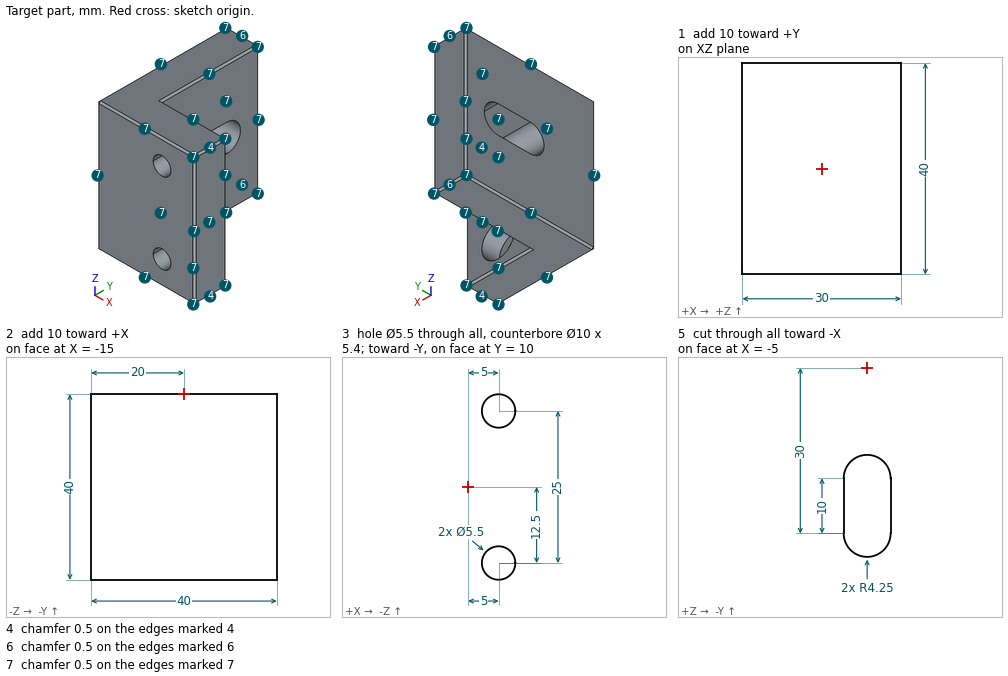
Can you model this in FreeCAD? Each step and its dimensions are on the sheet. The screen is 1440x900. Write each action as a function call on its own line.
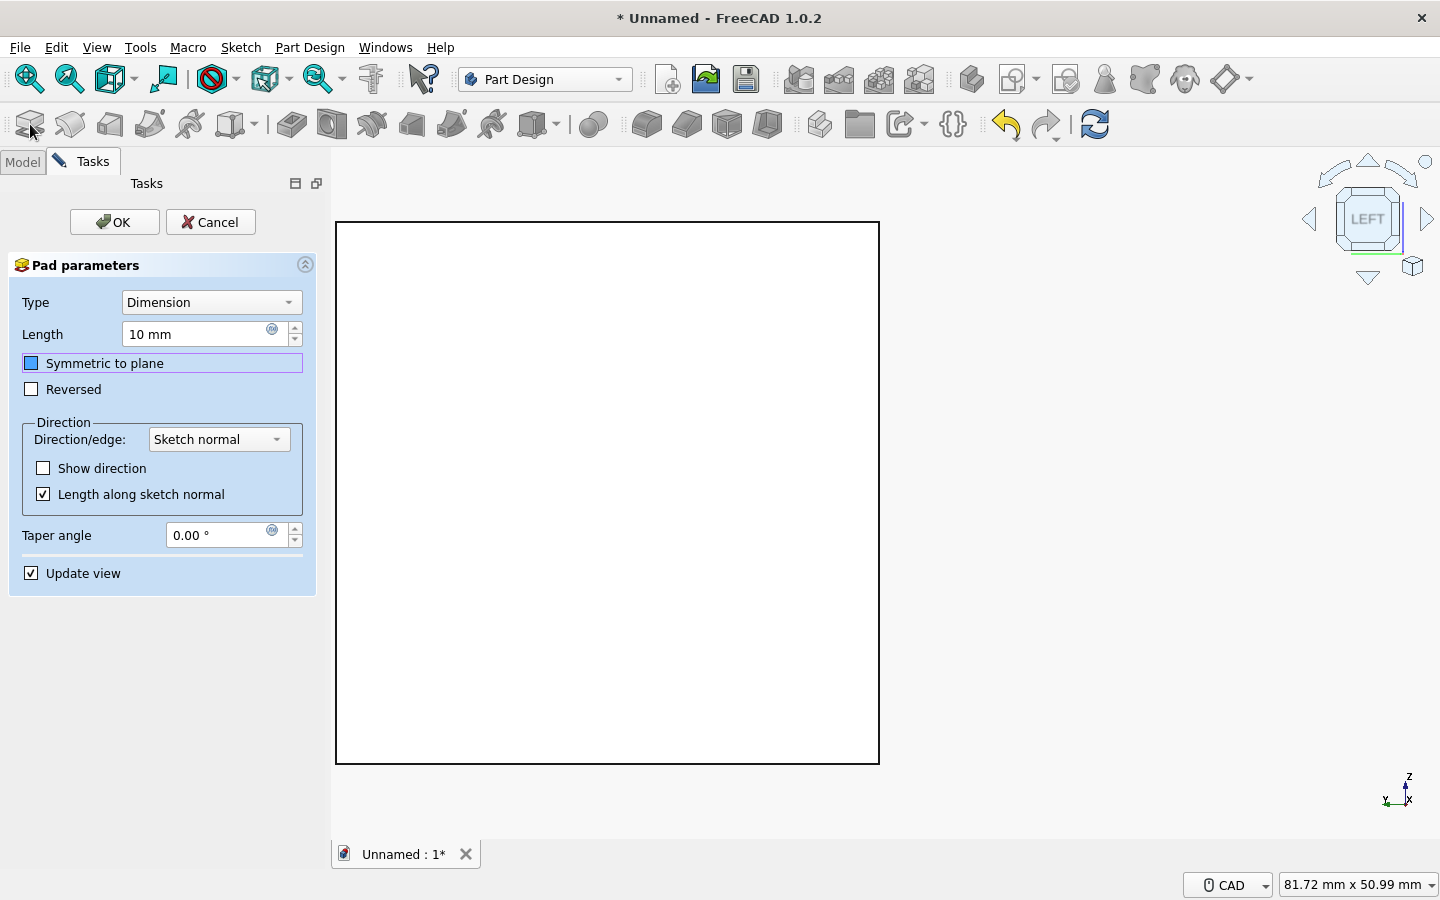
click(30, 389)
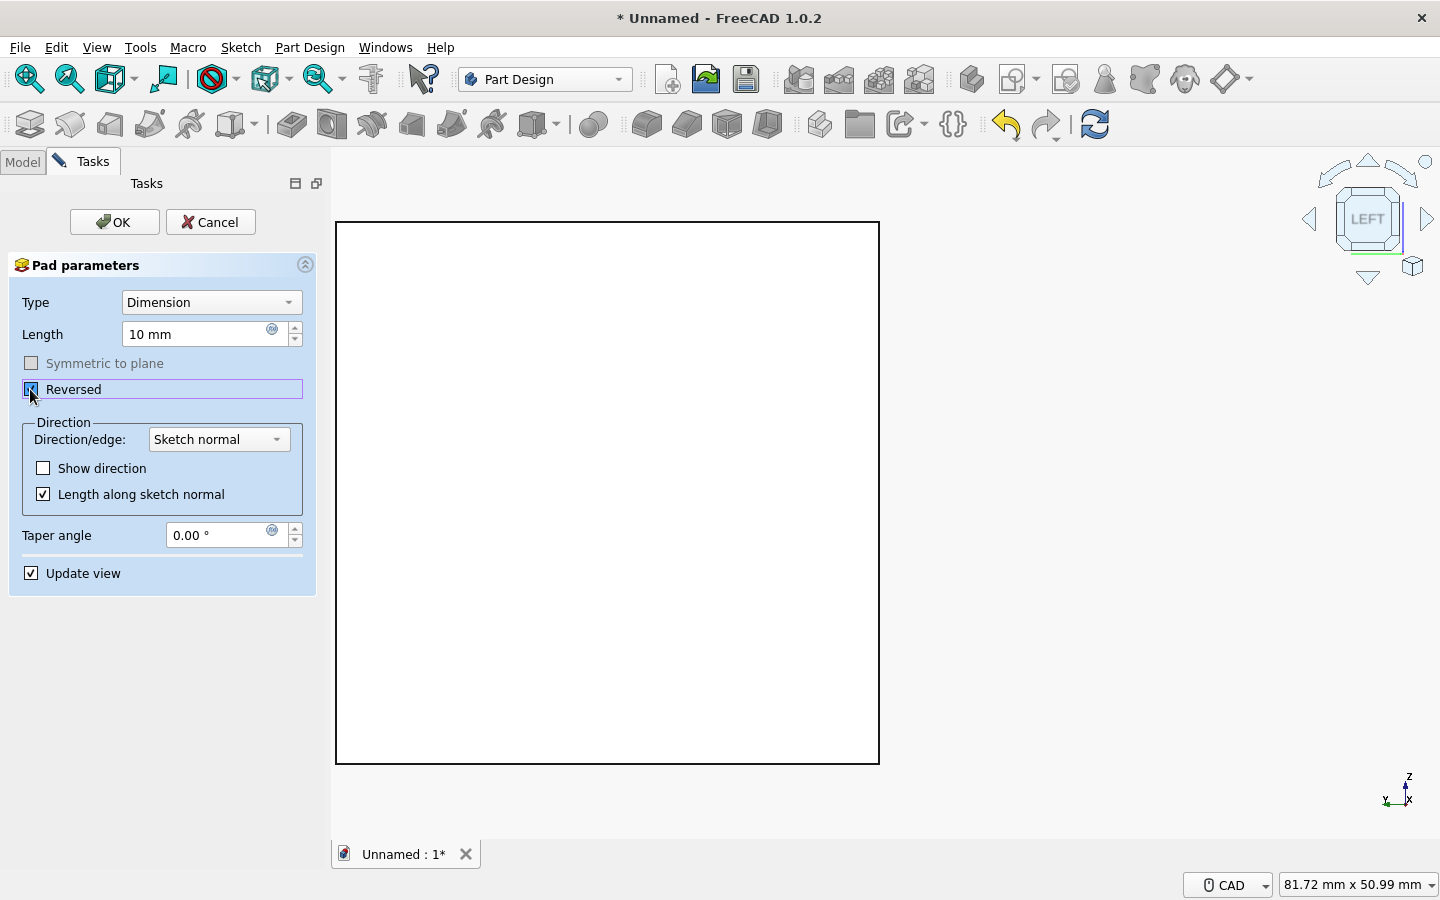
click(115, 222)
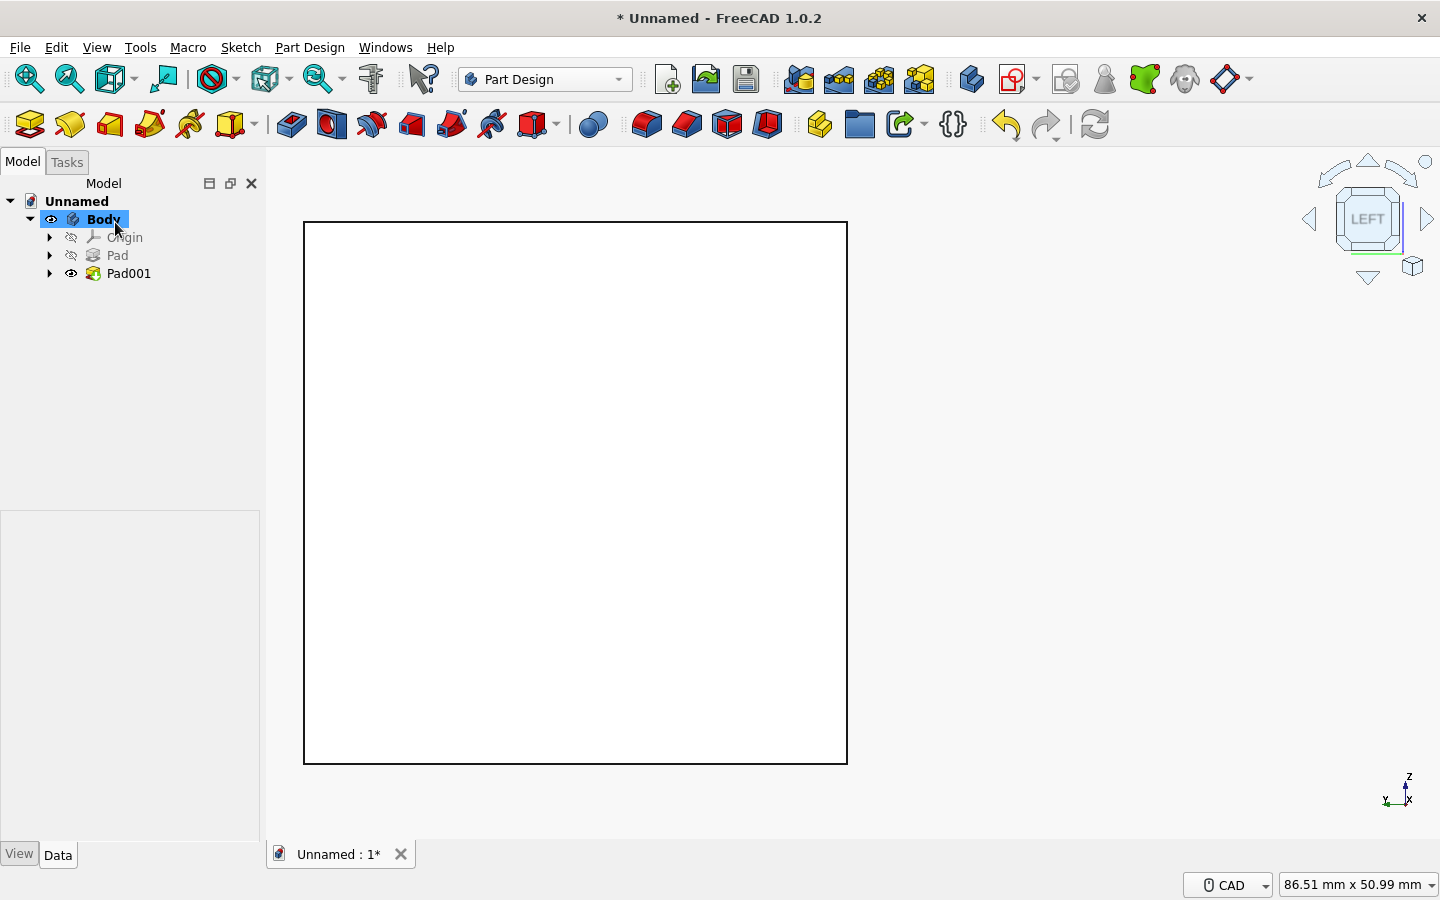
key(4)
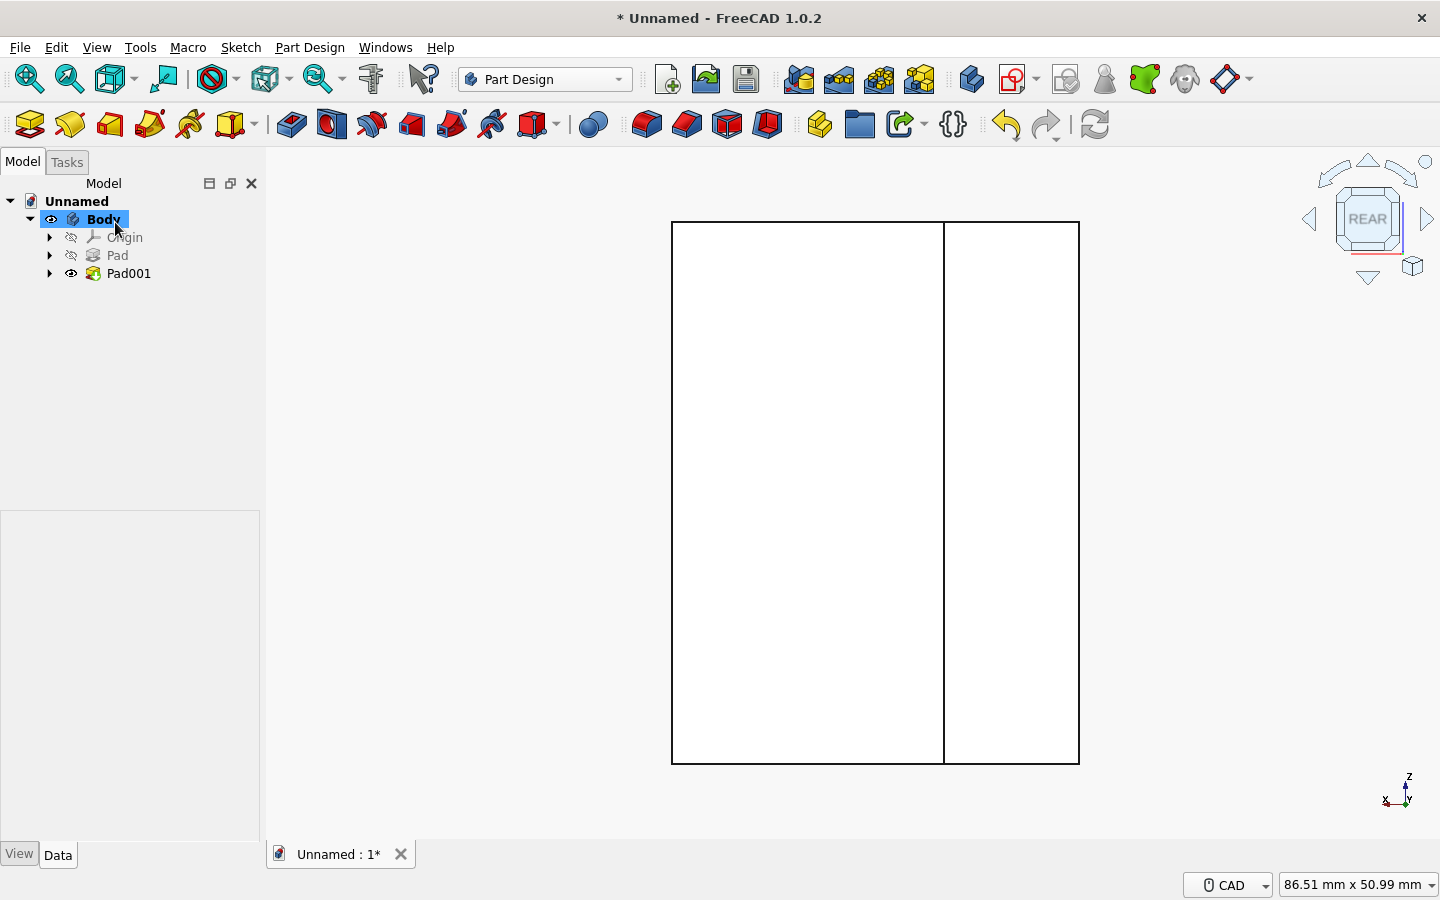
click(808, 414)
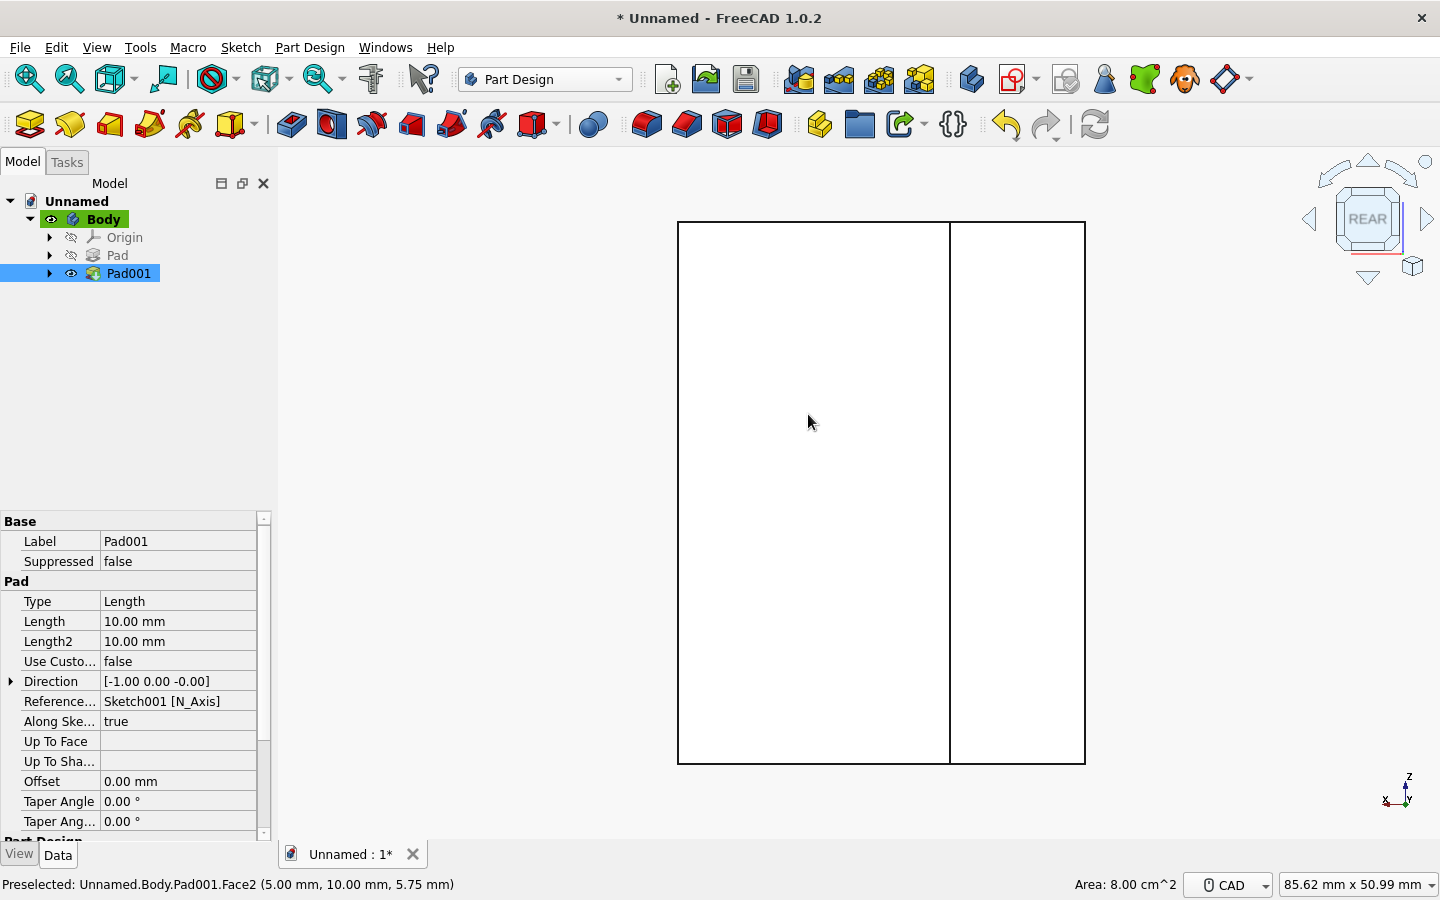
click(1012, 80)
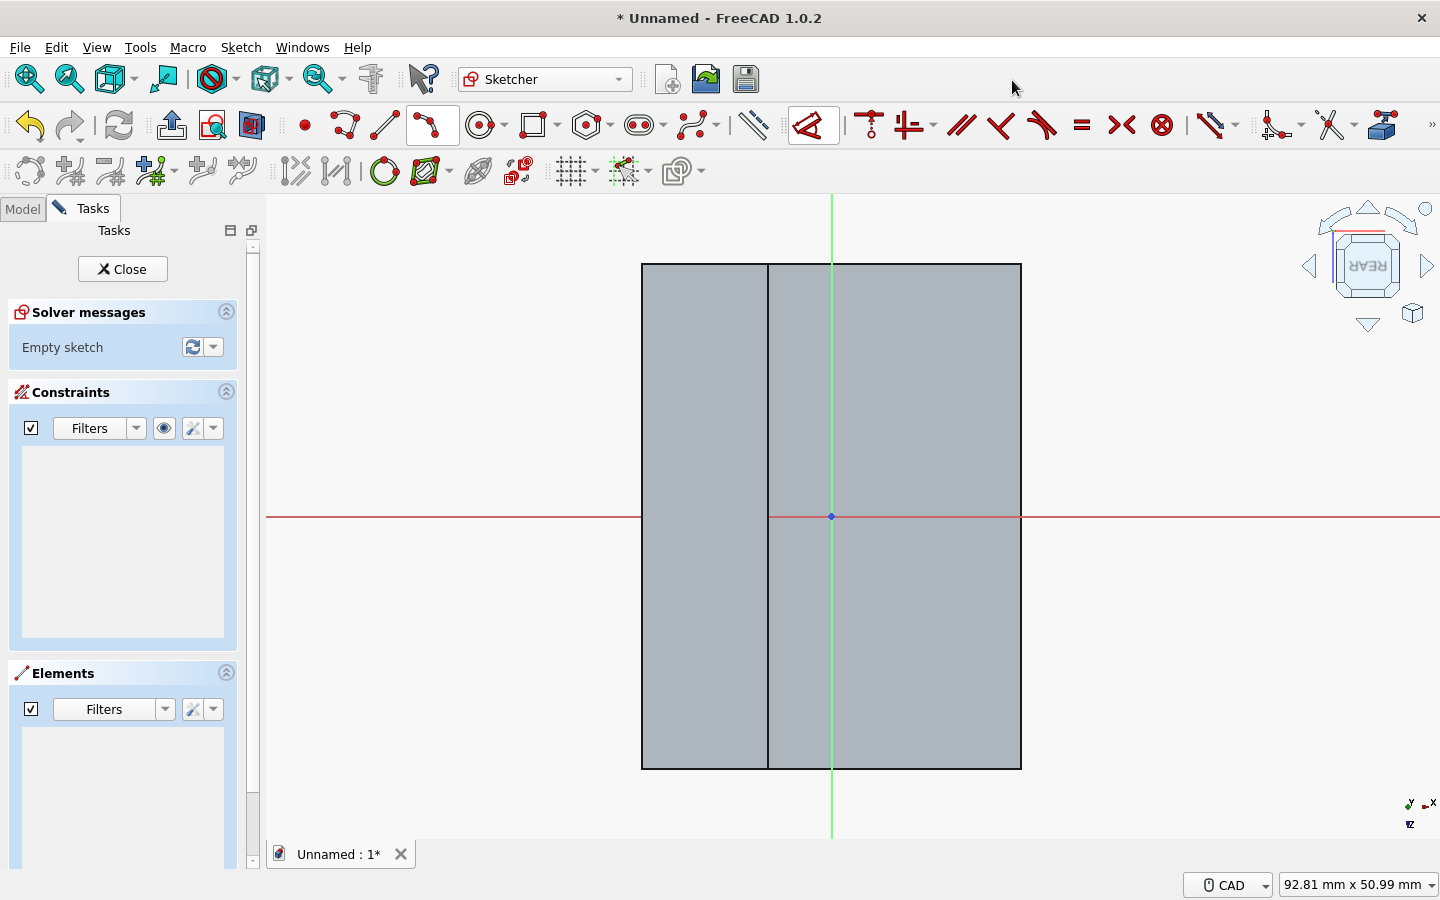
click(252, 126)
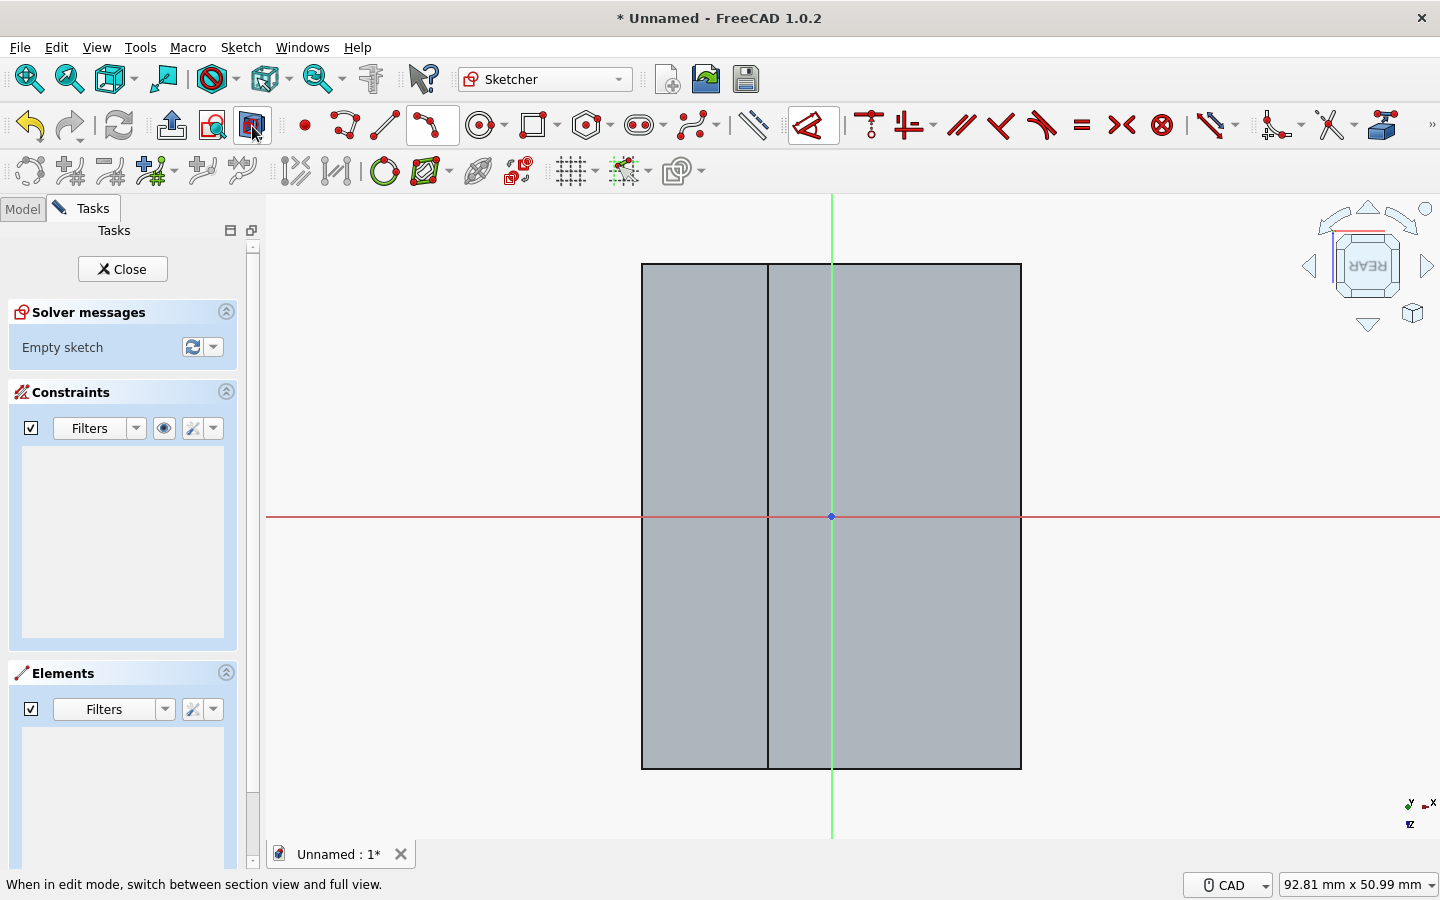
click(480, 126)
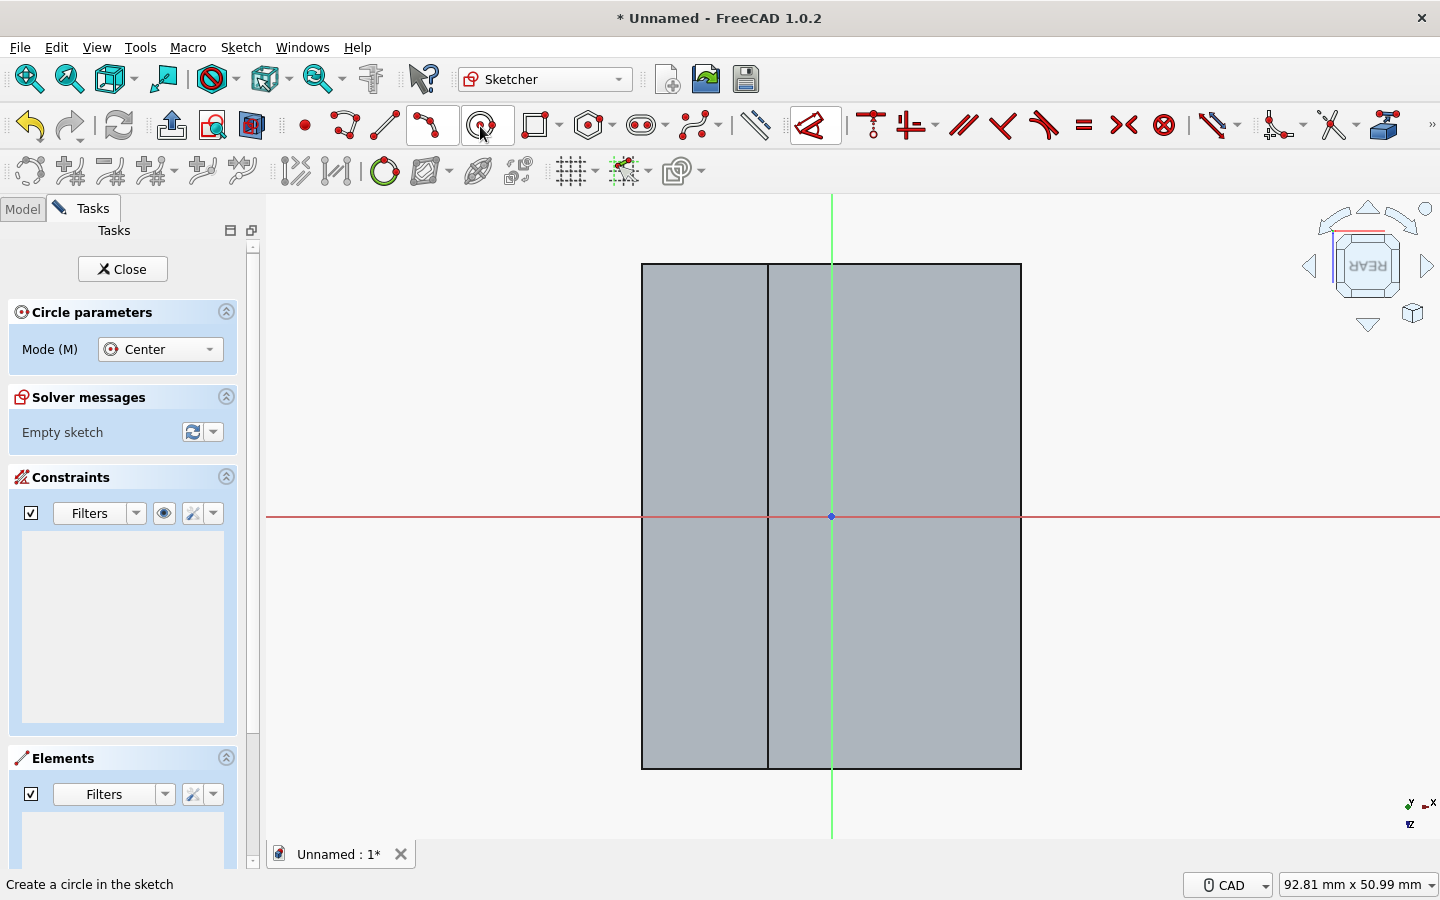
click(895, 675)
click(920, 650)